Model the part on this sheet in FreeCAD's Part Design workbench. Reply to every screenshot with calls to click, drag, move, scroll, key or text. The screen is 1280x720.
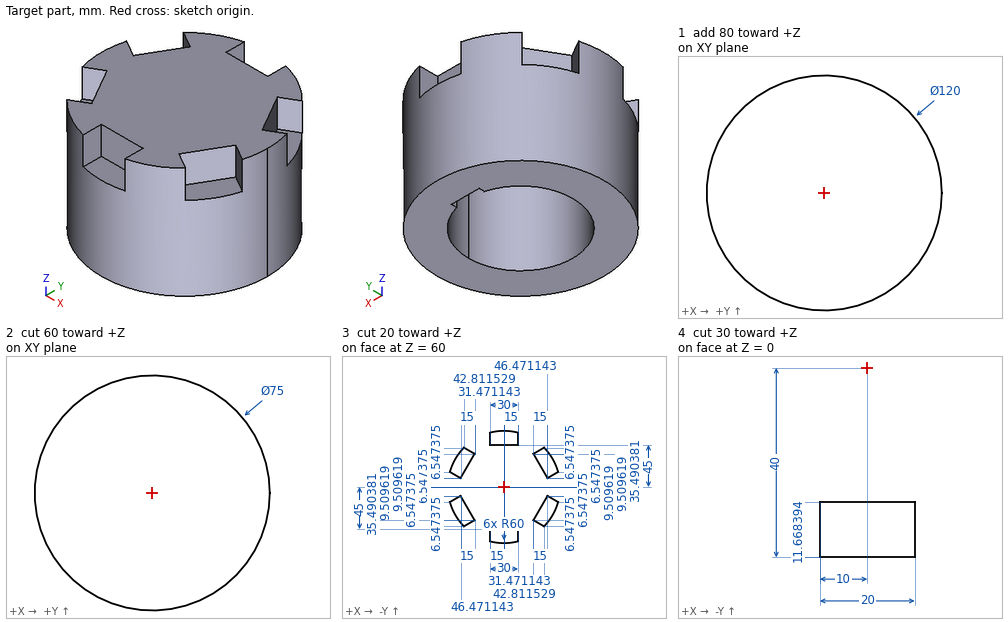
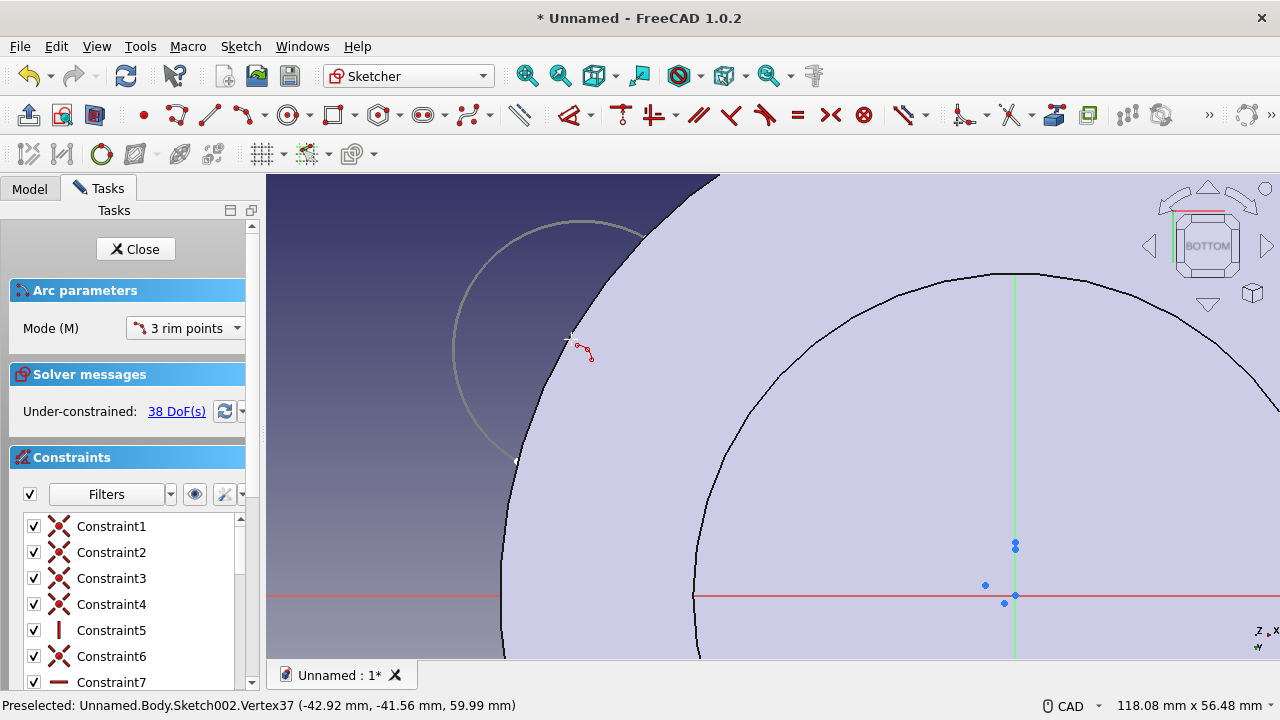
click(569, 338)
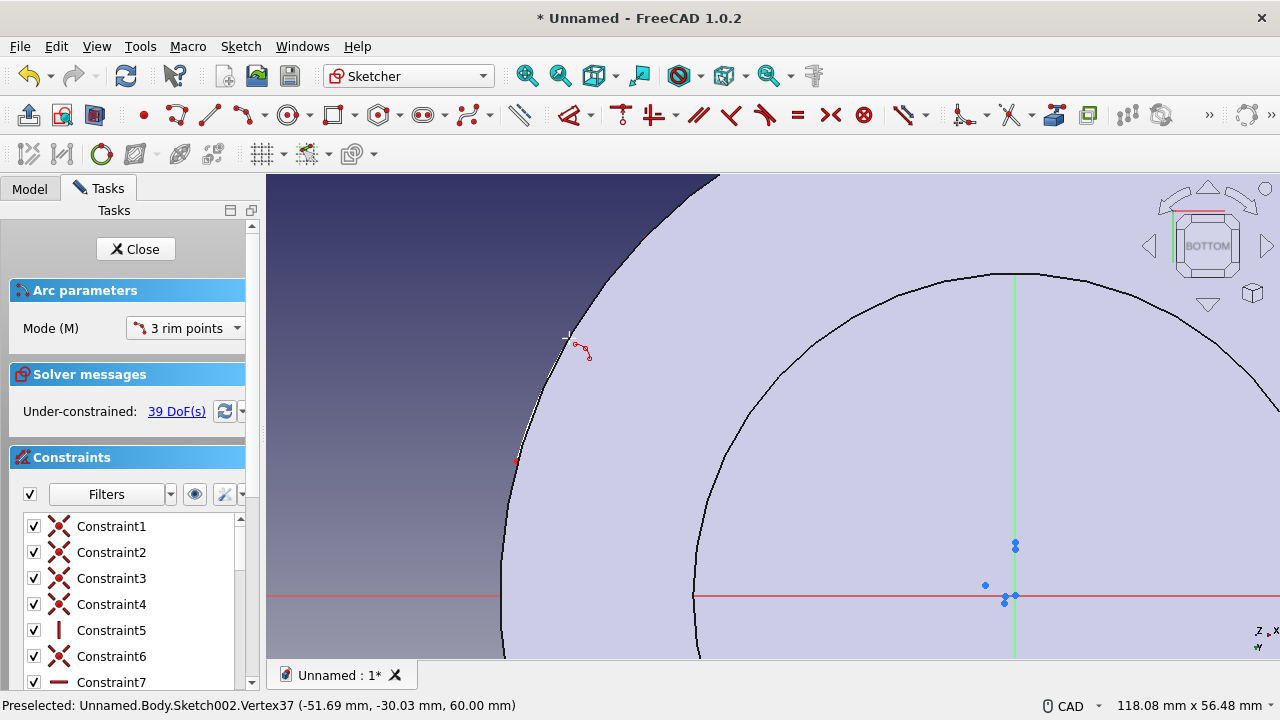
click(177, 116)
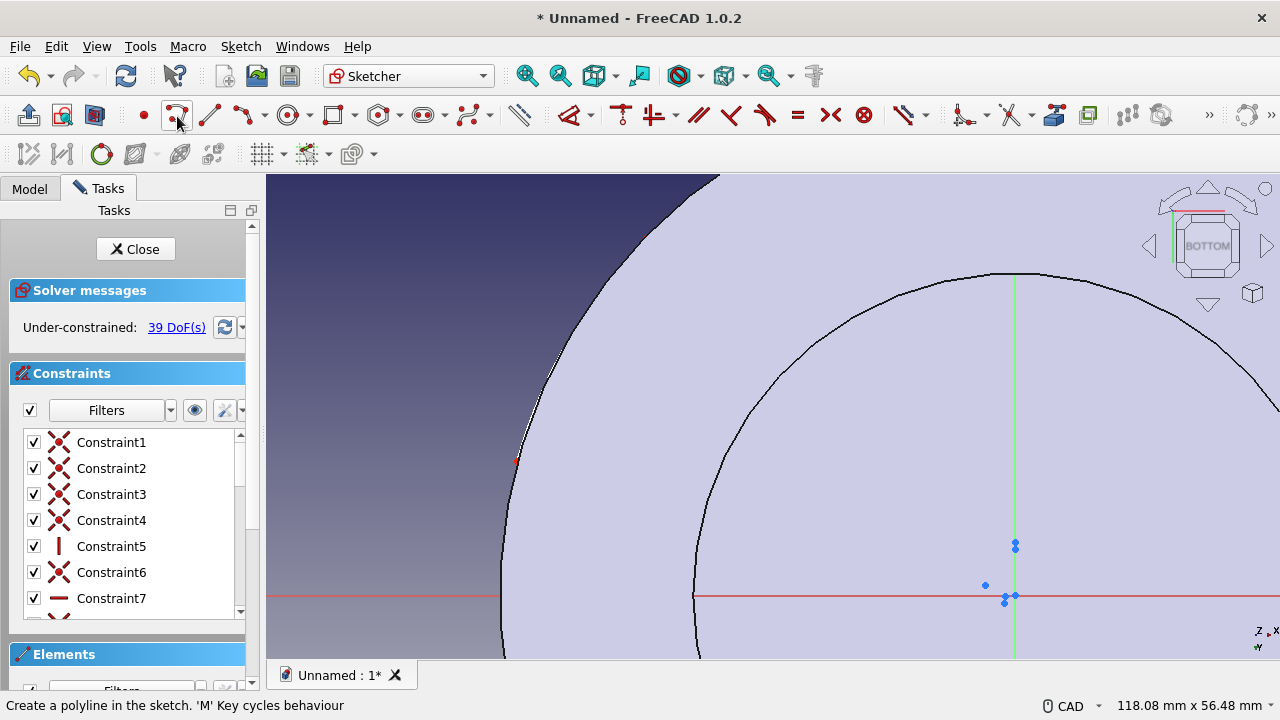
scroll(571, 339, down, 6)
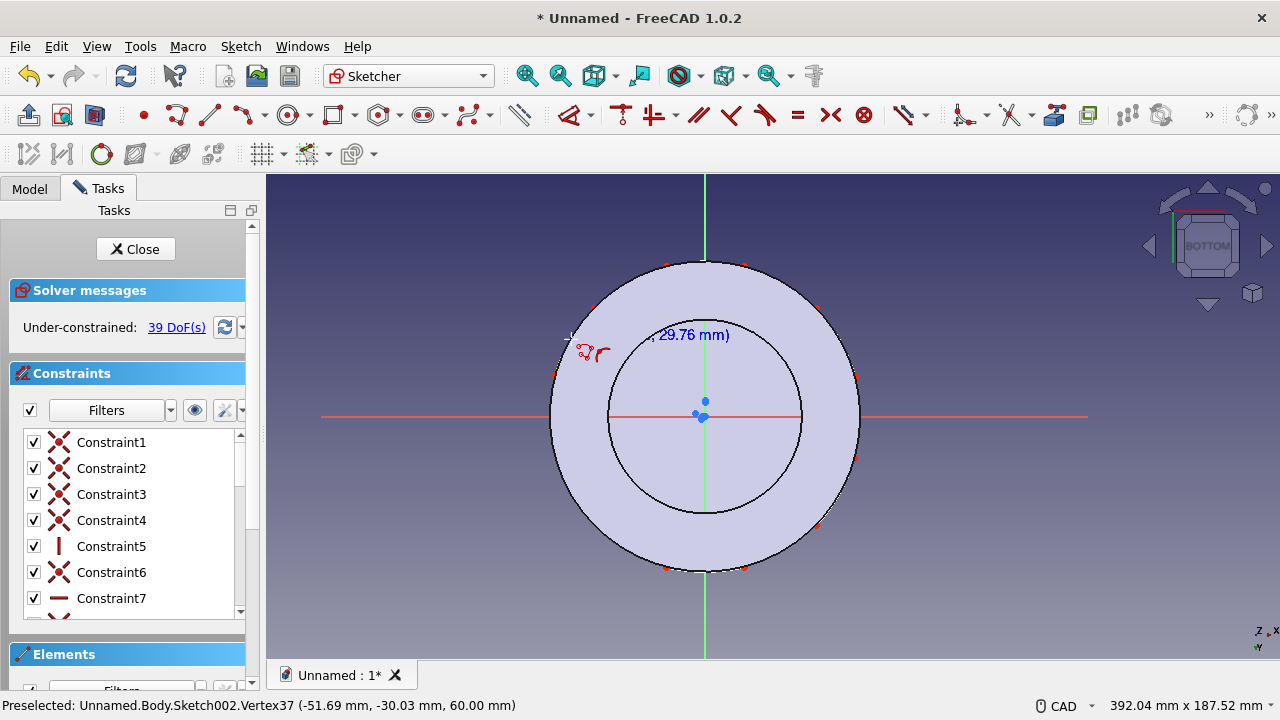
click(555, 458)
click(585, 441)
click(624, 508)
click(594, 525)
right_click(594, 525)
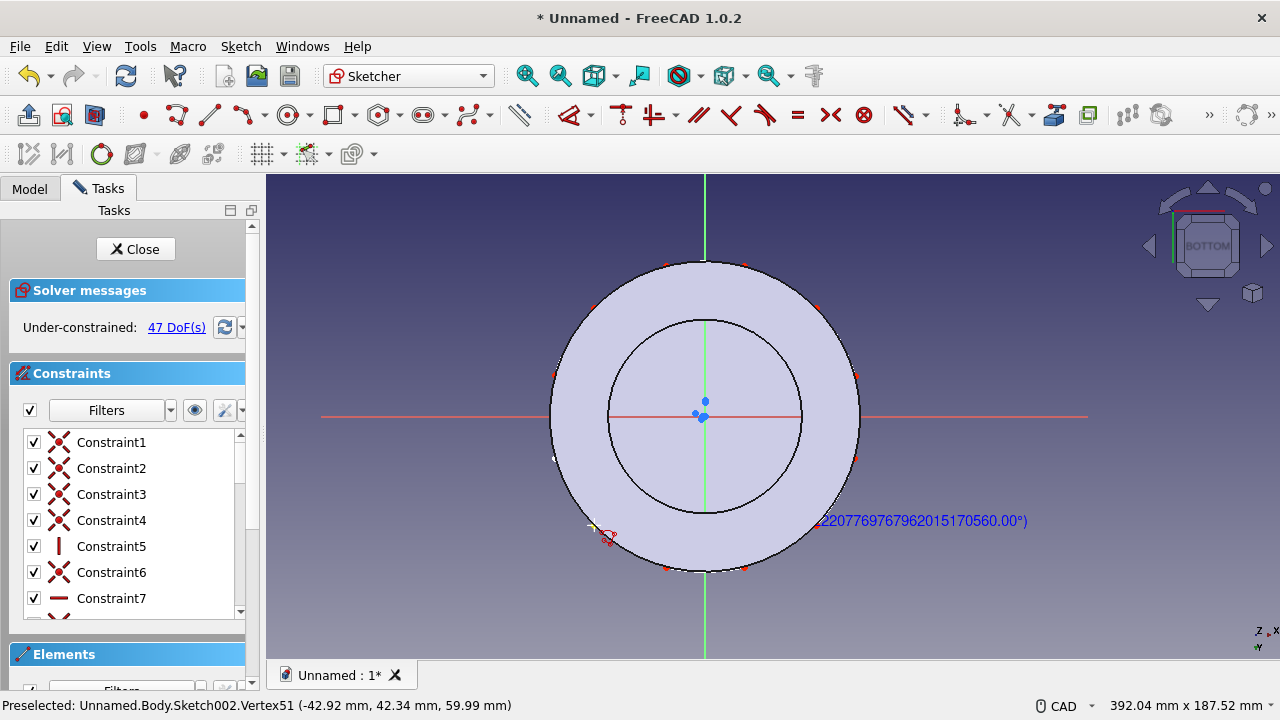
click(242, 116)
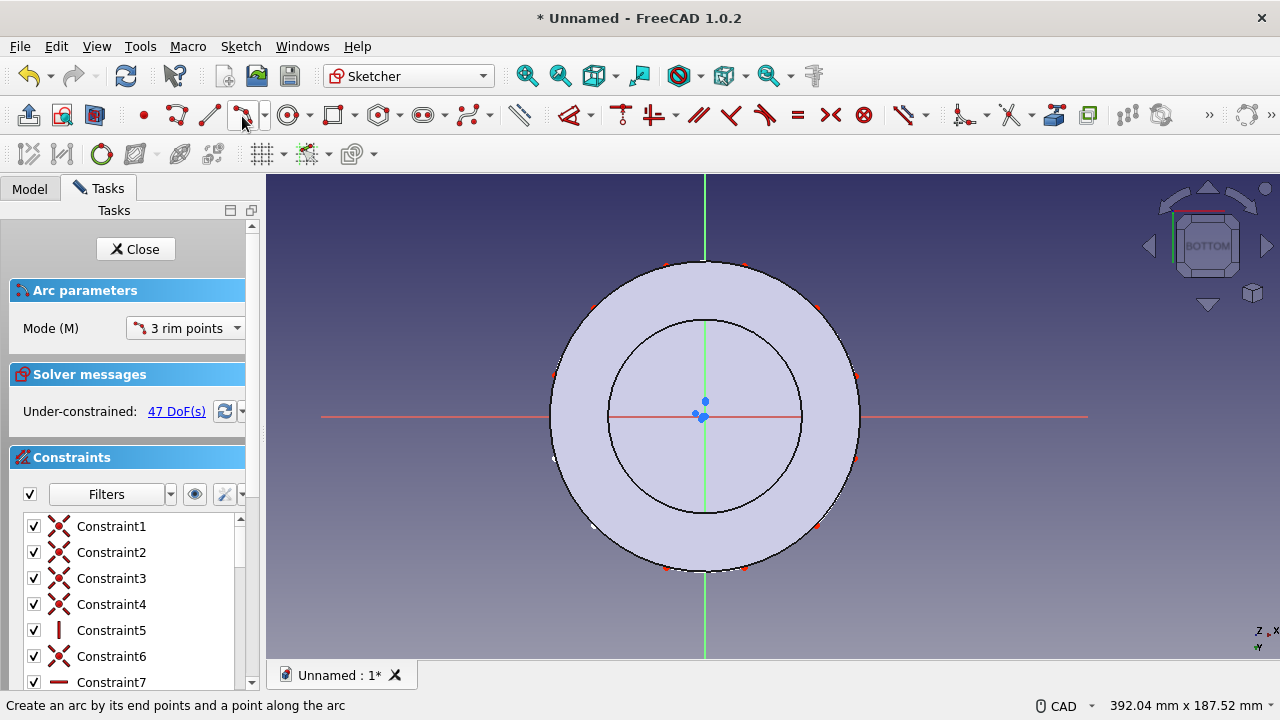
click(594, 526)
click(555, 459)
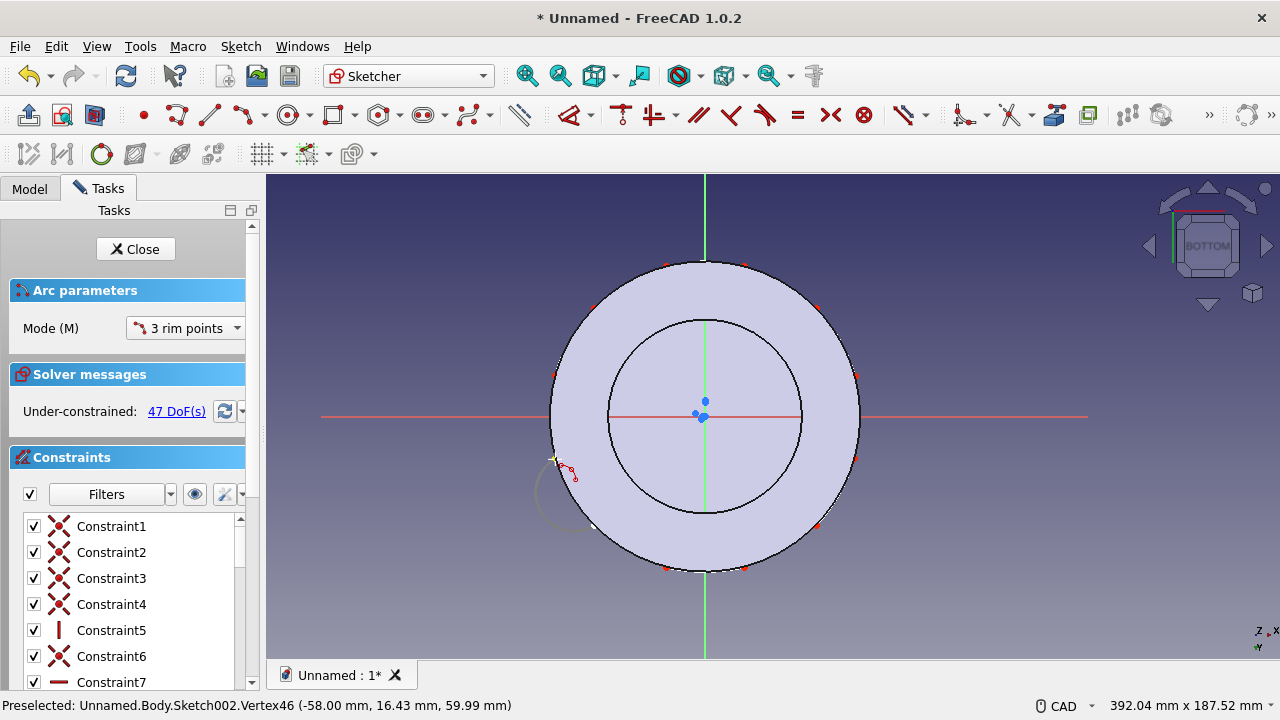
scroll(571, 494, up, 6)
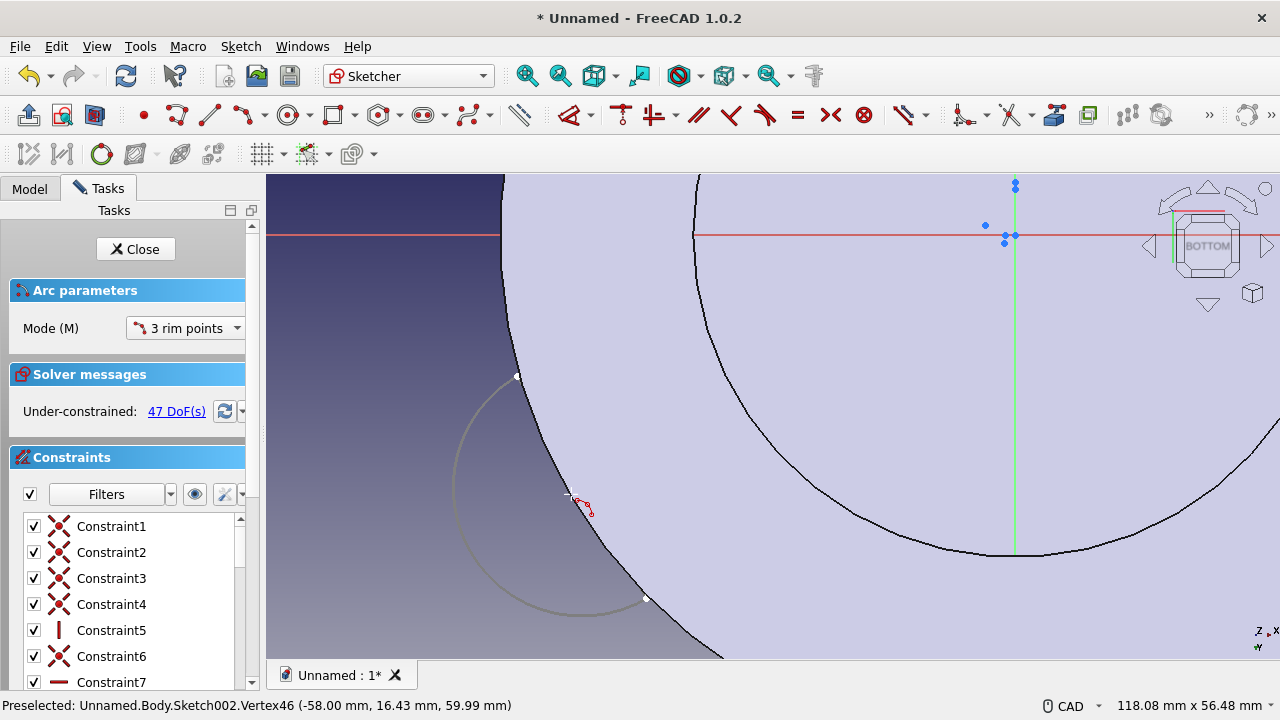
click(569, 493)
key(Escape)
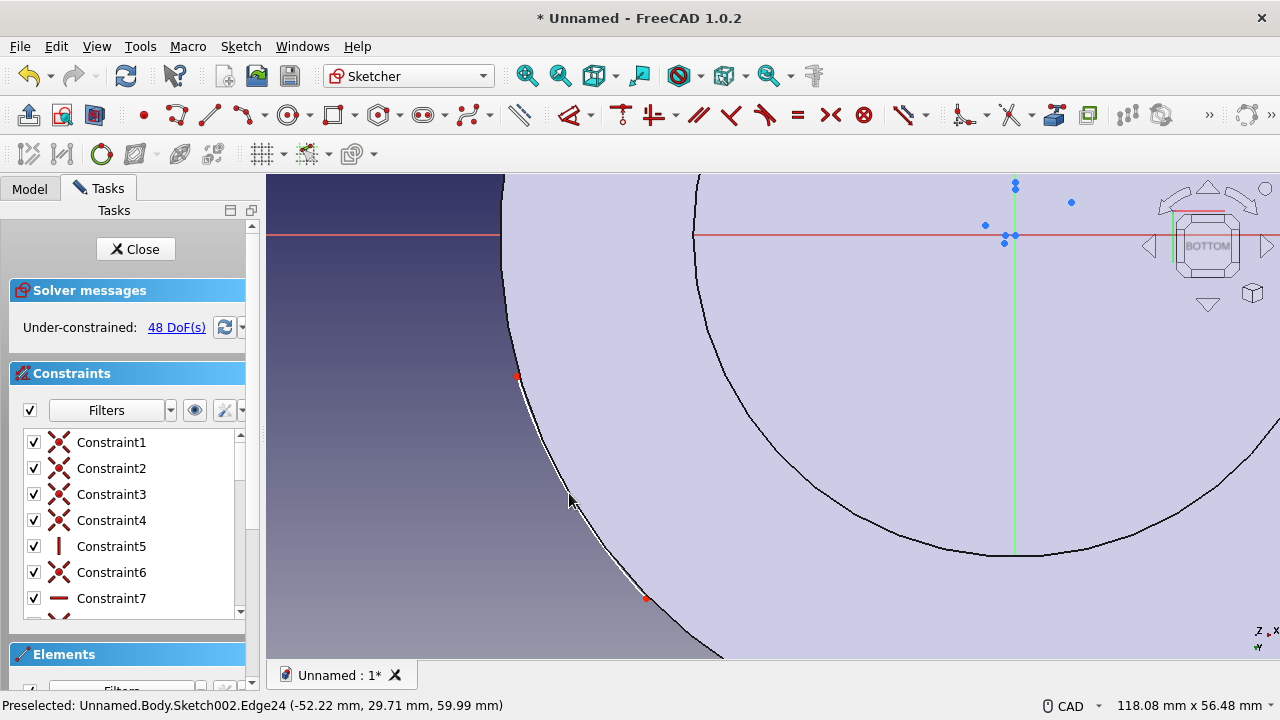
scroll(571, 495, down, 6)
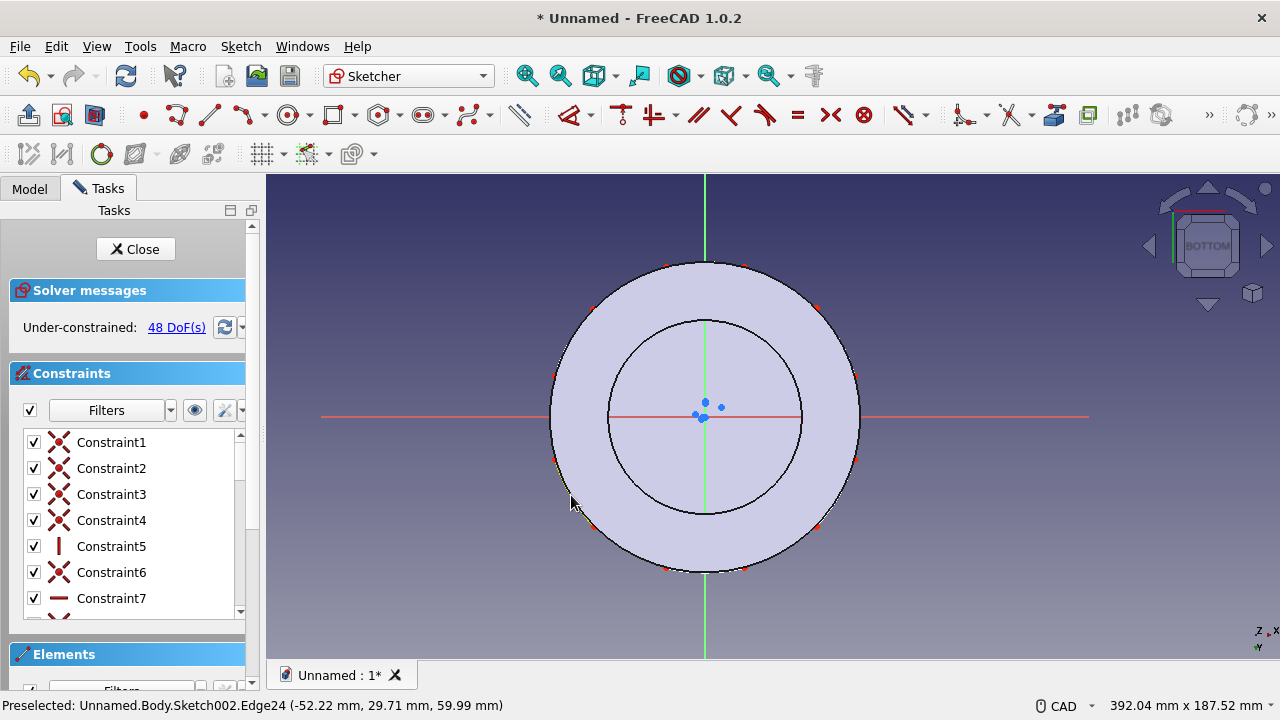
click(831, 509)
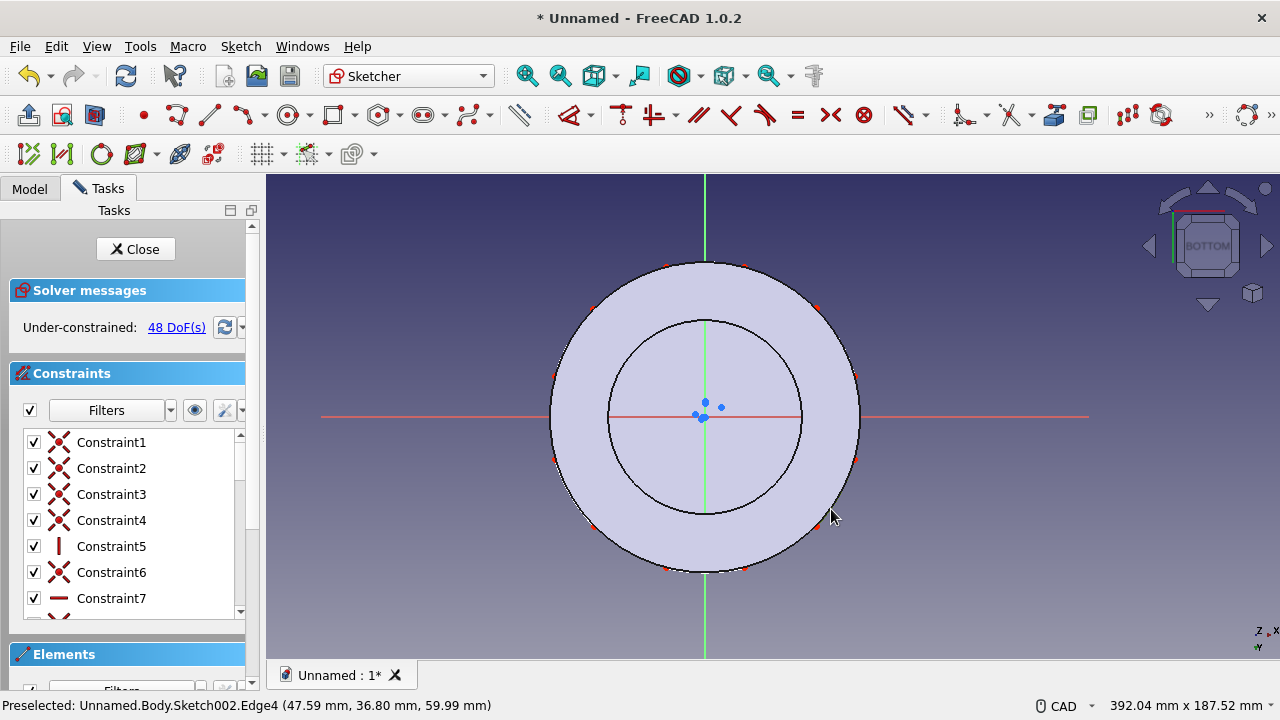
click(689, 572)